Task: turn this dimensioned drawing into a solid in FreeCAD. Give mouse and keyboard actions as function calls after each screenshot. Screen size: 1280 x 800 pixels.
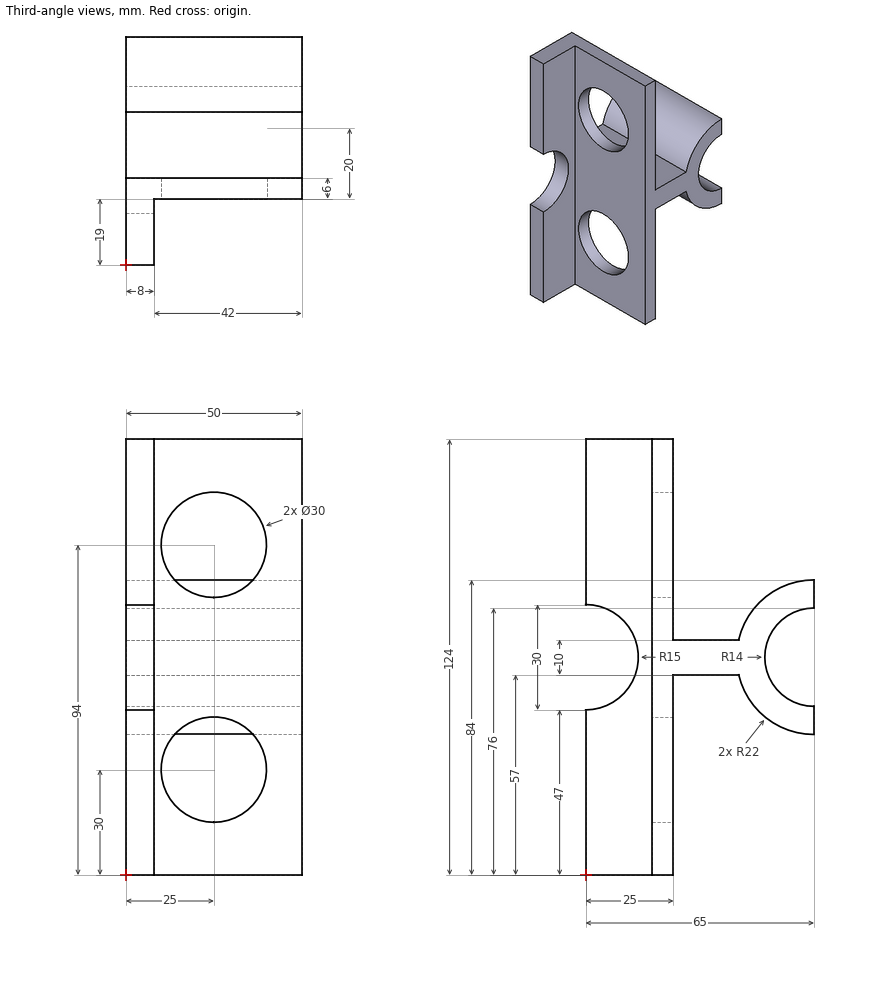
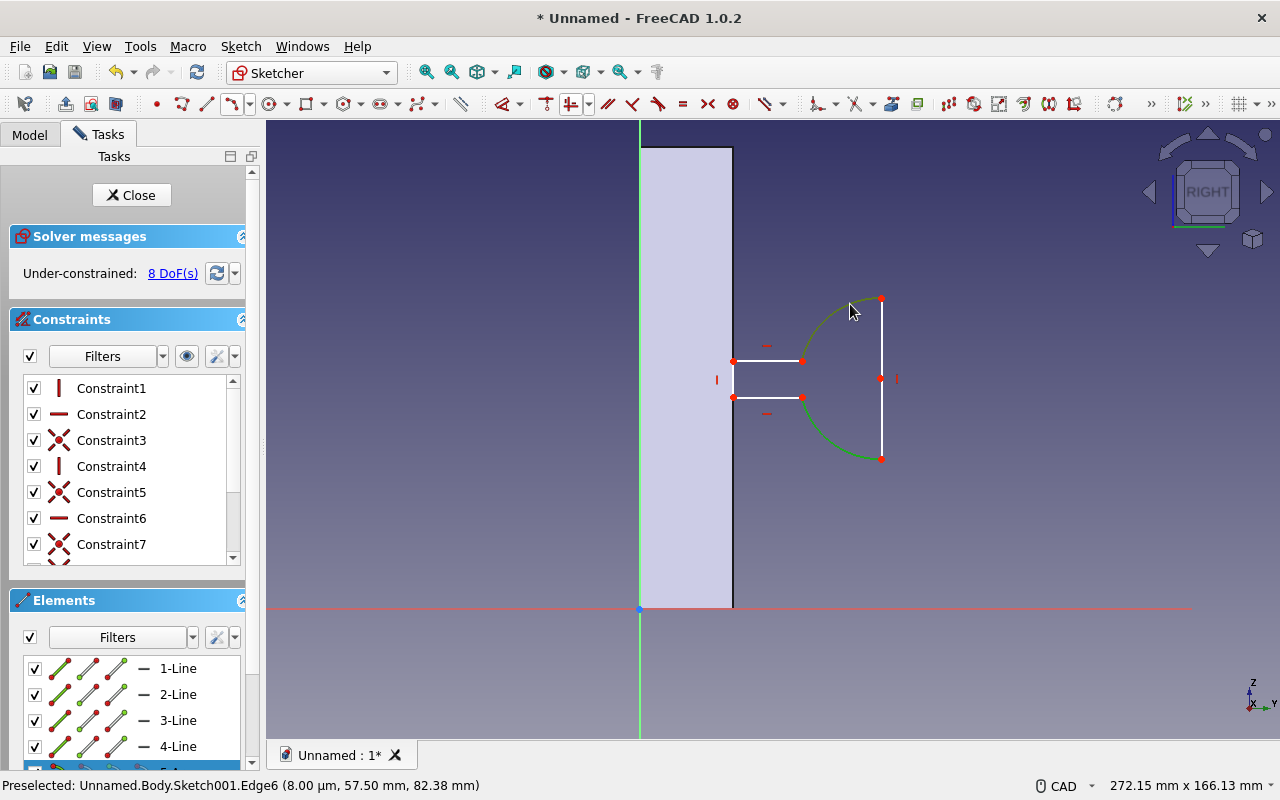
key(e)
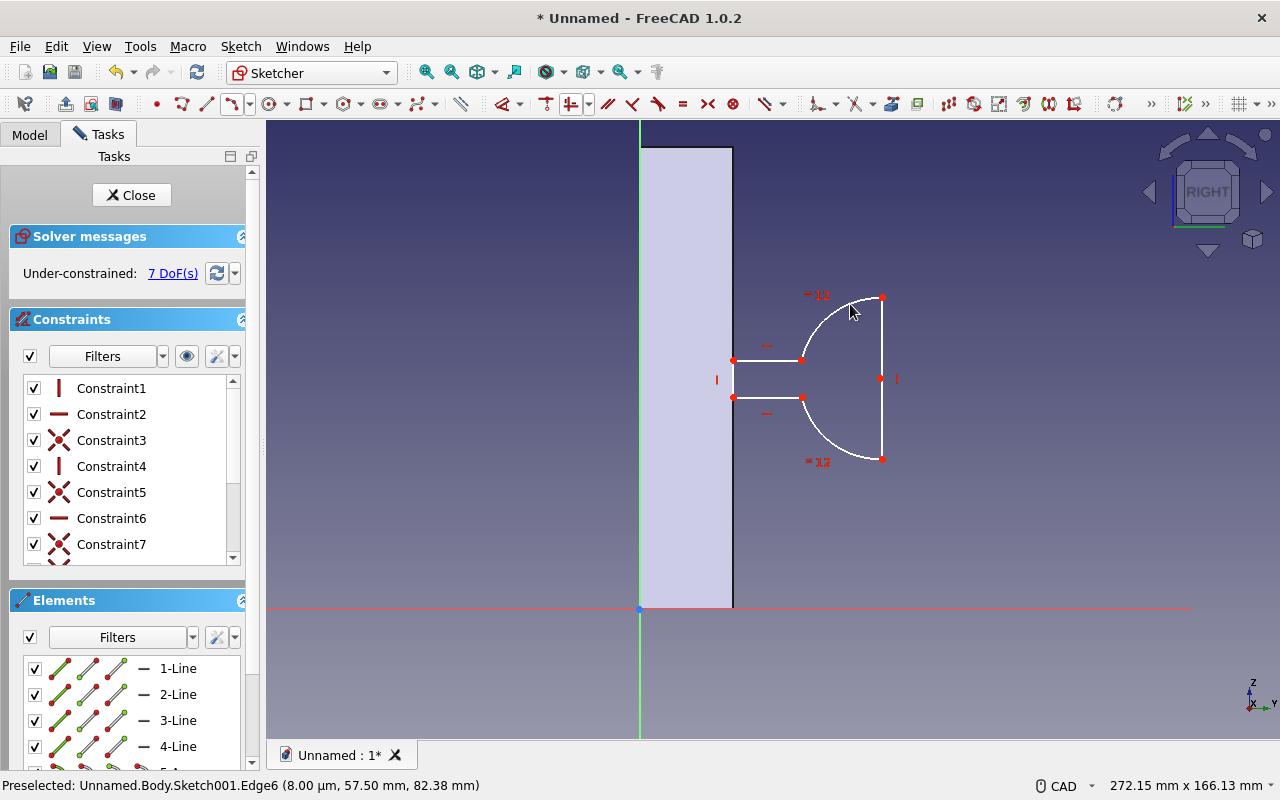
key(d)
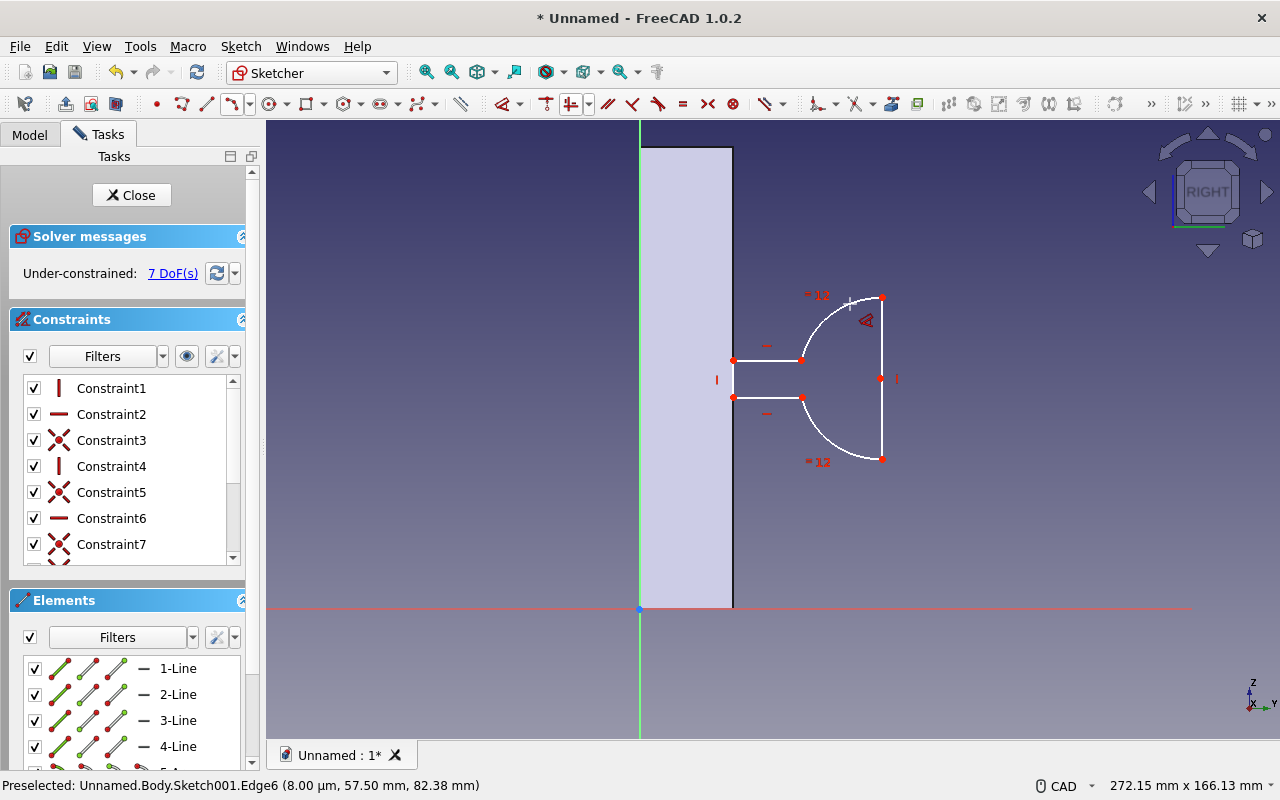
click(816, 427)
click(790, 446)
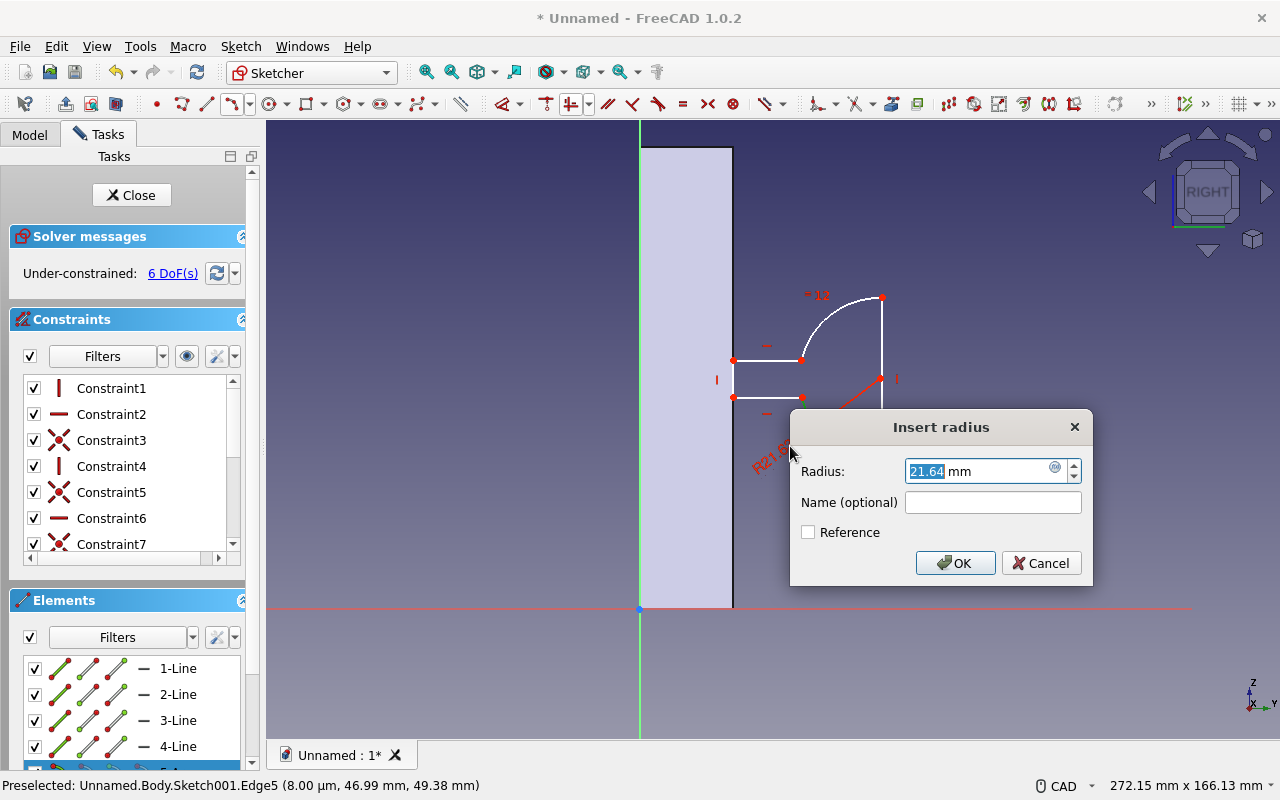
text(22)
key(Return)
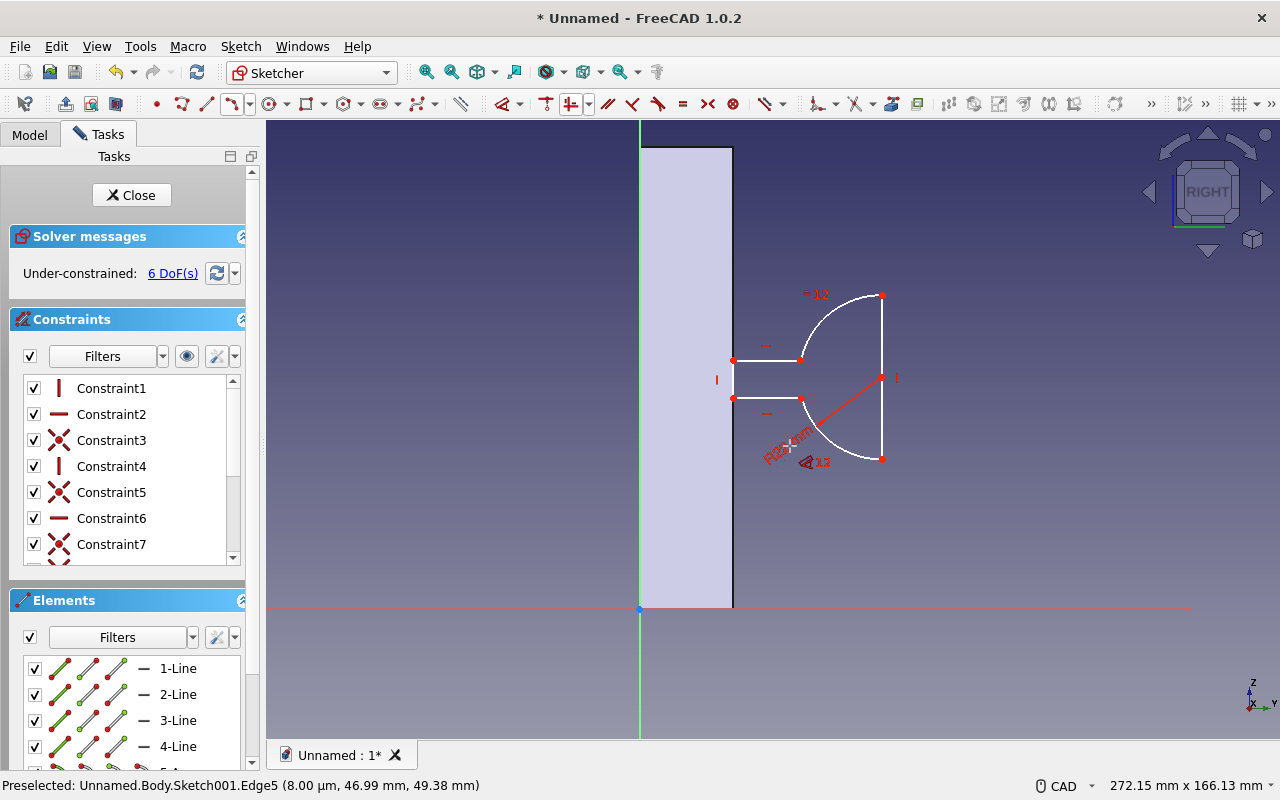
scroll(733, 387, up, 2)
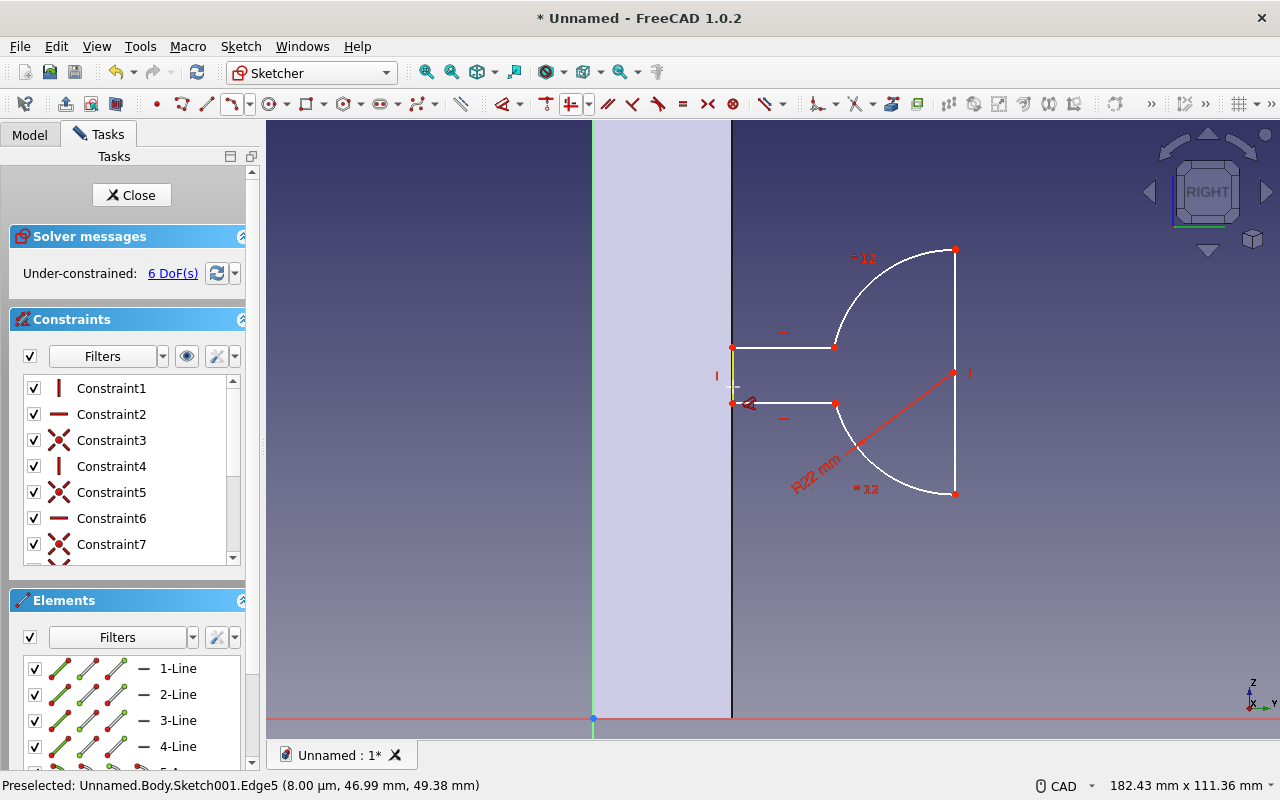
click(733, 387)
click(699, 376)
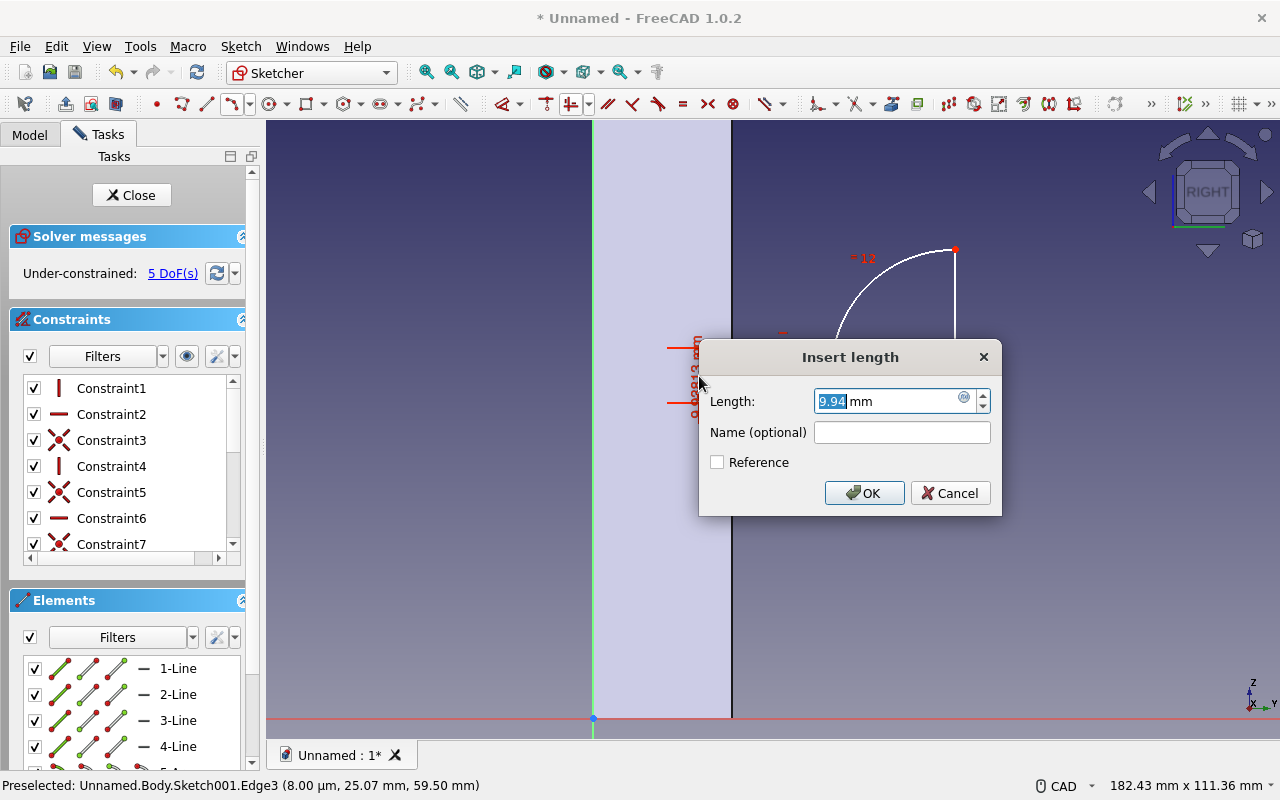
text(10)
key(Return)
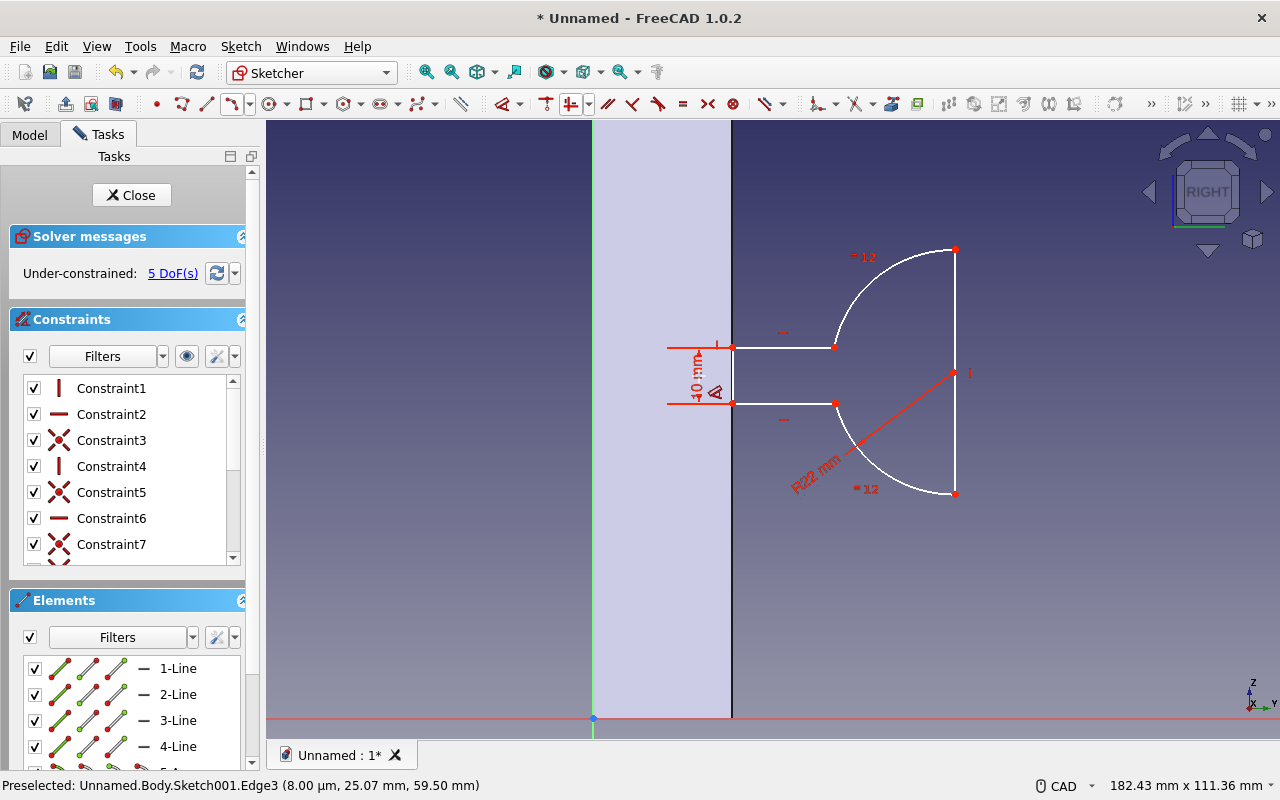
click(955, 250)
click(774, 216)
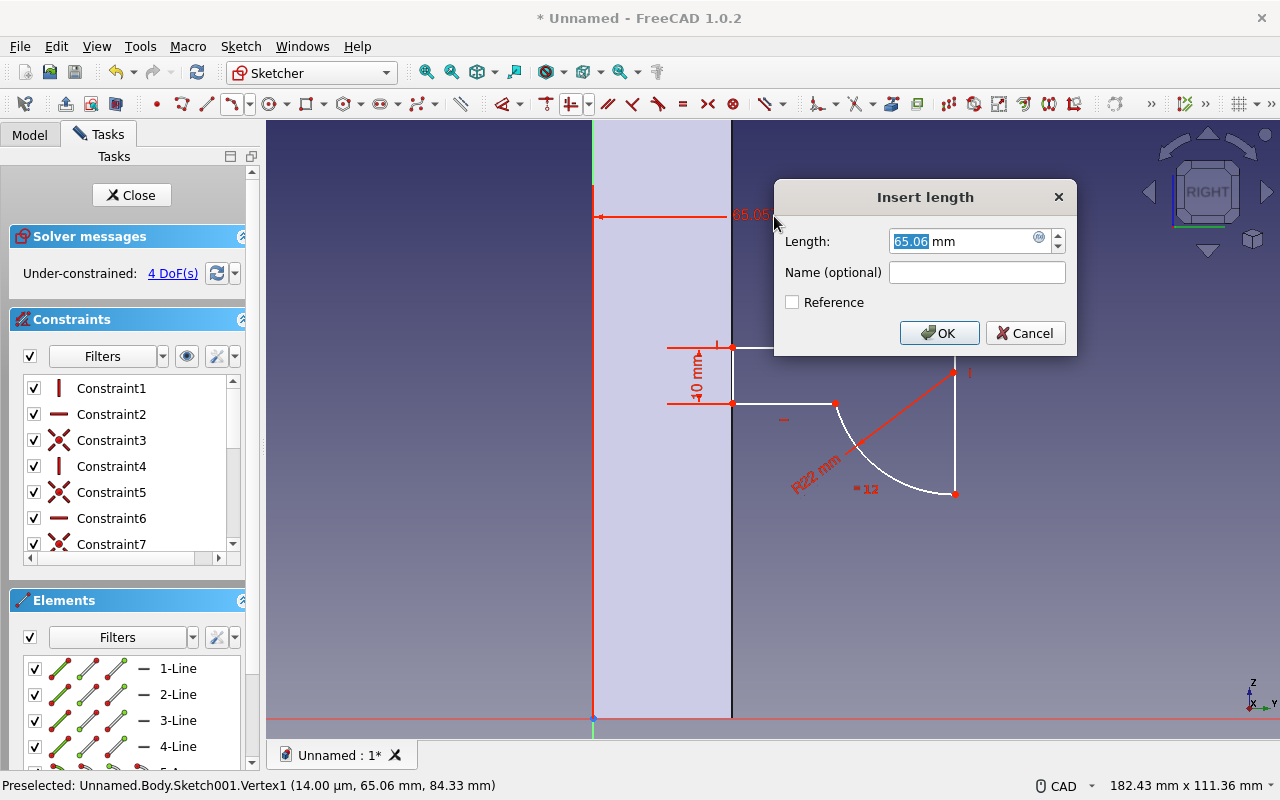
text(65)
key(Return)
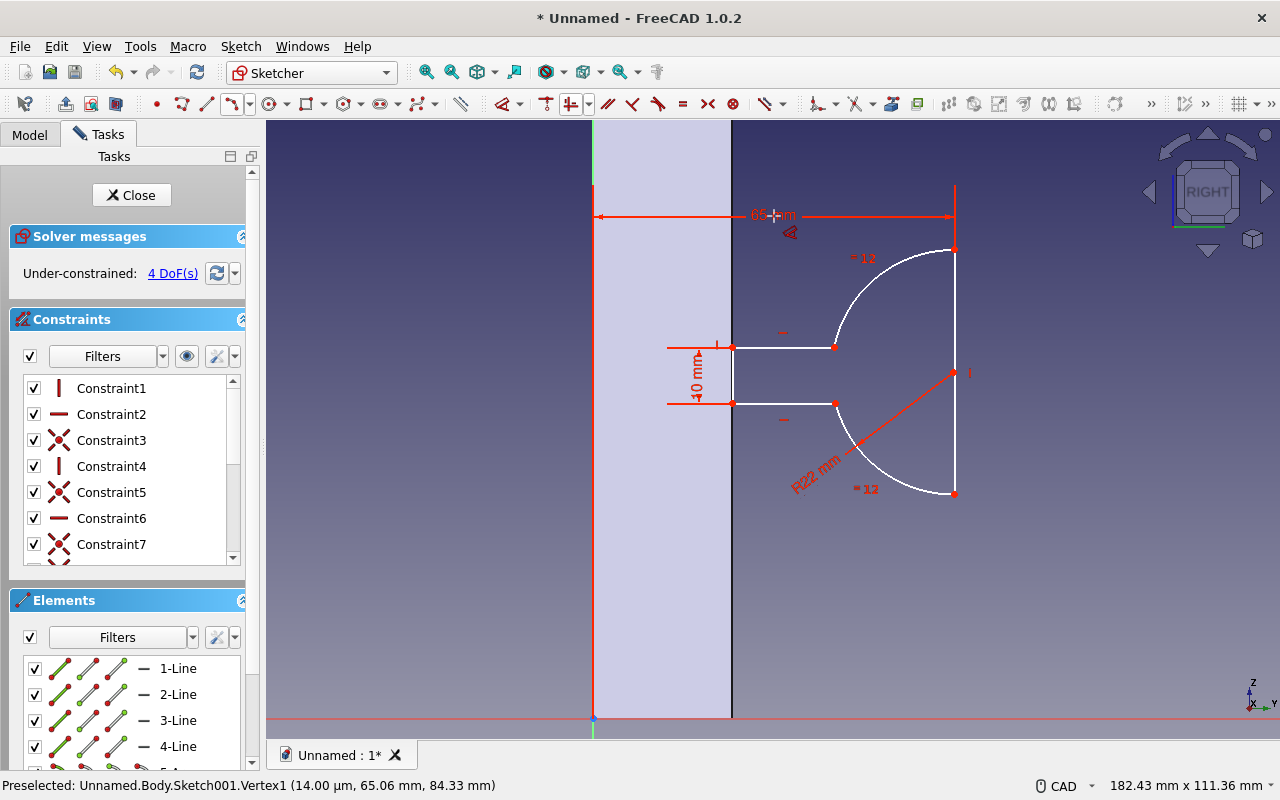
click(955, 250)
click(989, 480)